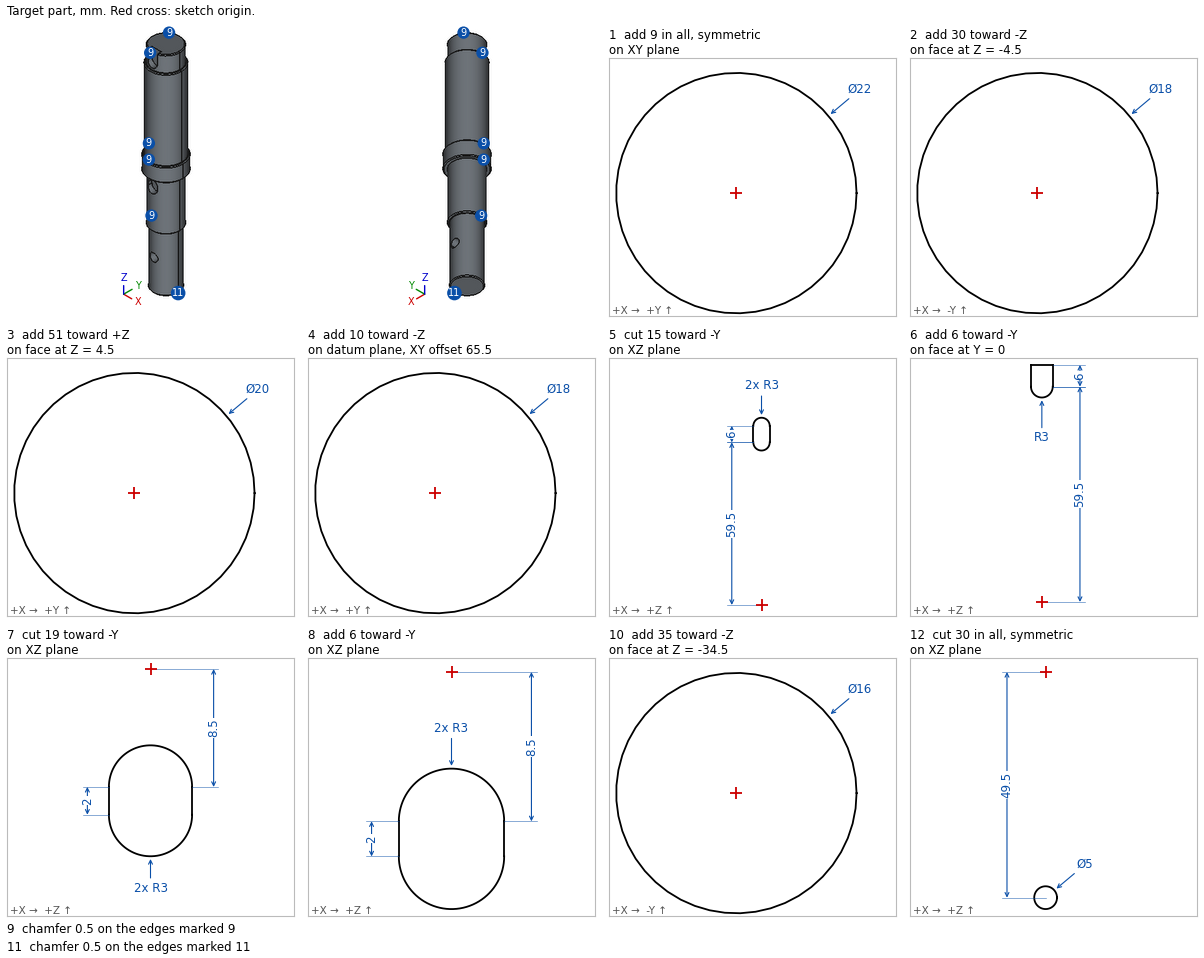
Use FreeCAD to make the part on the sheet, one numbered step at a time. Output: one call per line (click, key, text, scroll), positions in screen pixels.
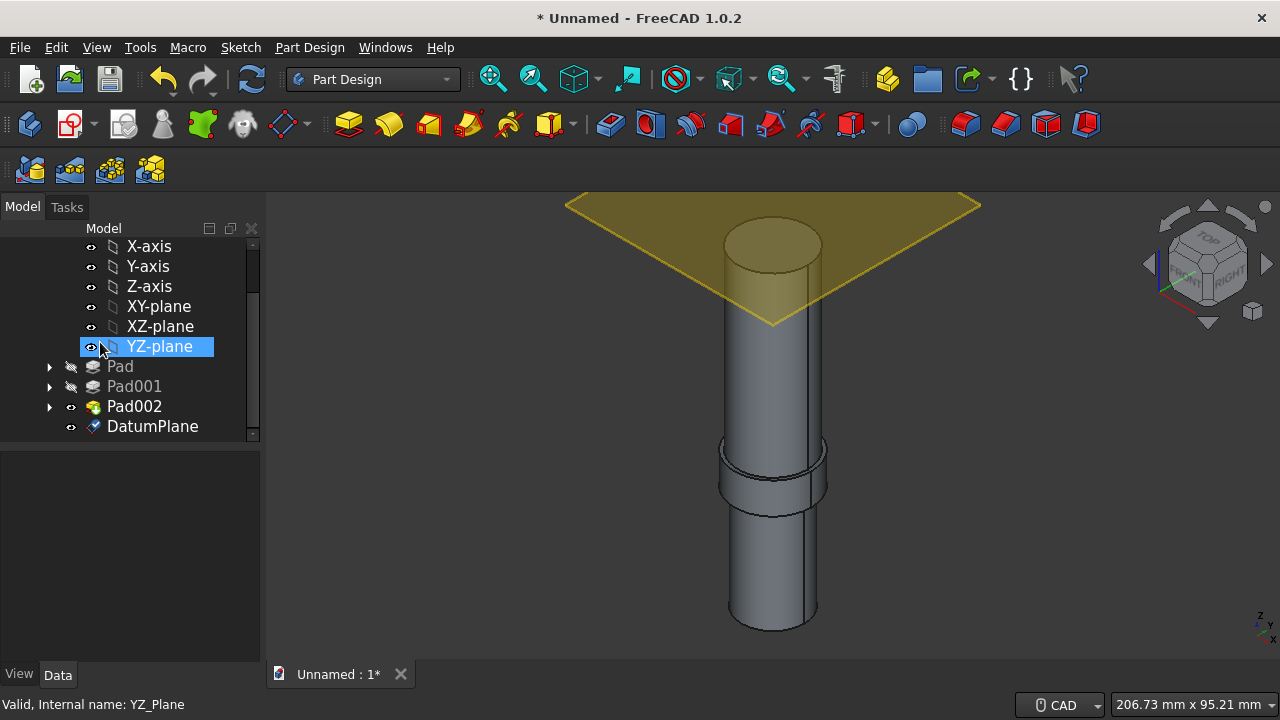
click(116, 427)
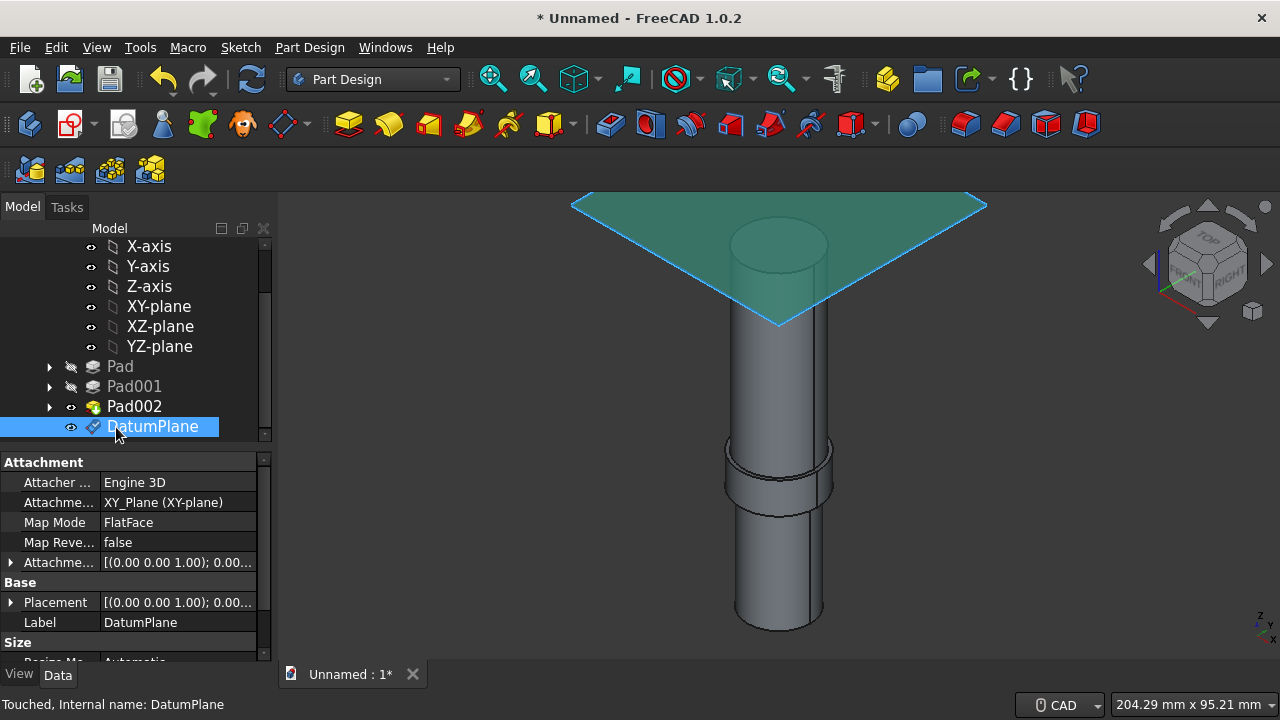
click(70, 124)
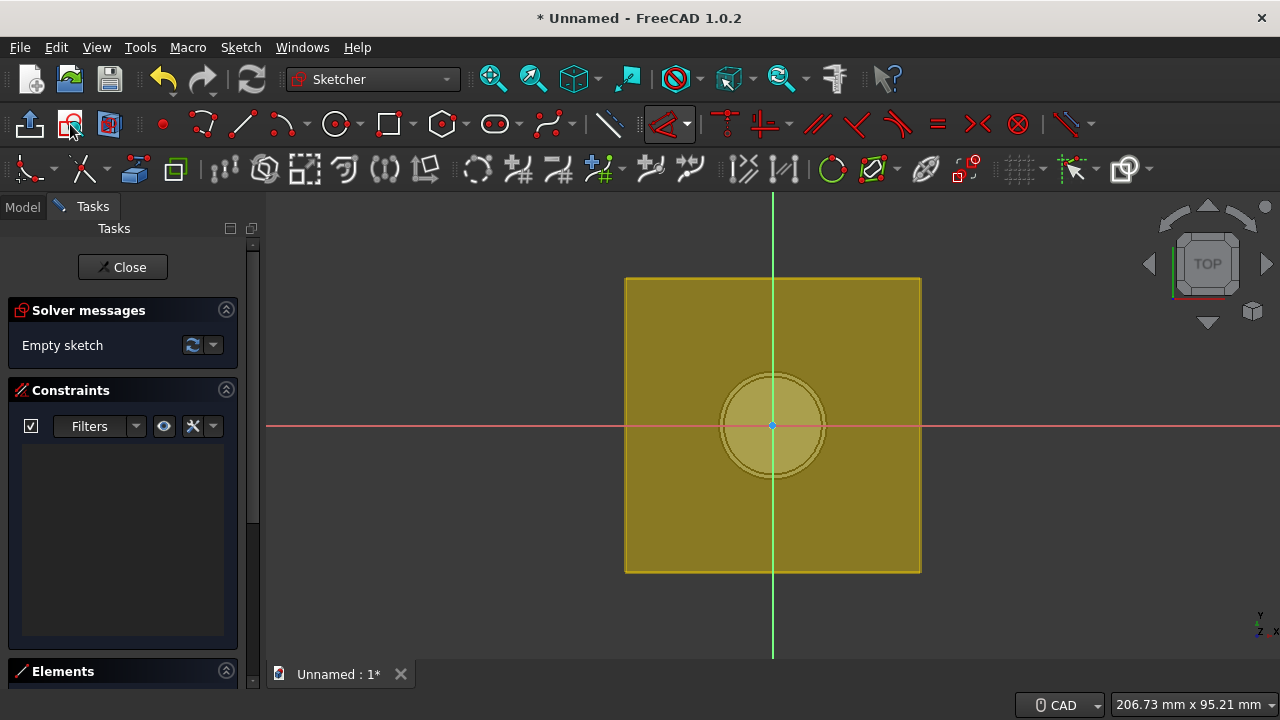
scroll(802, 426, up, 6)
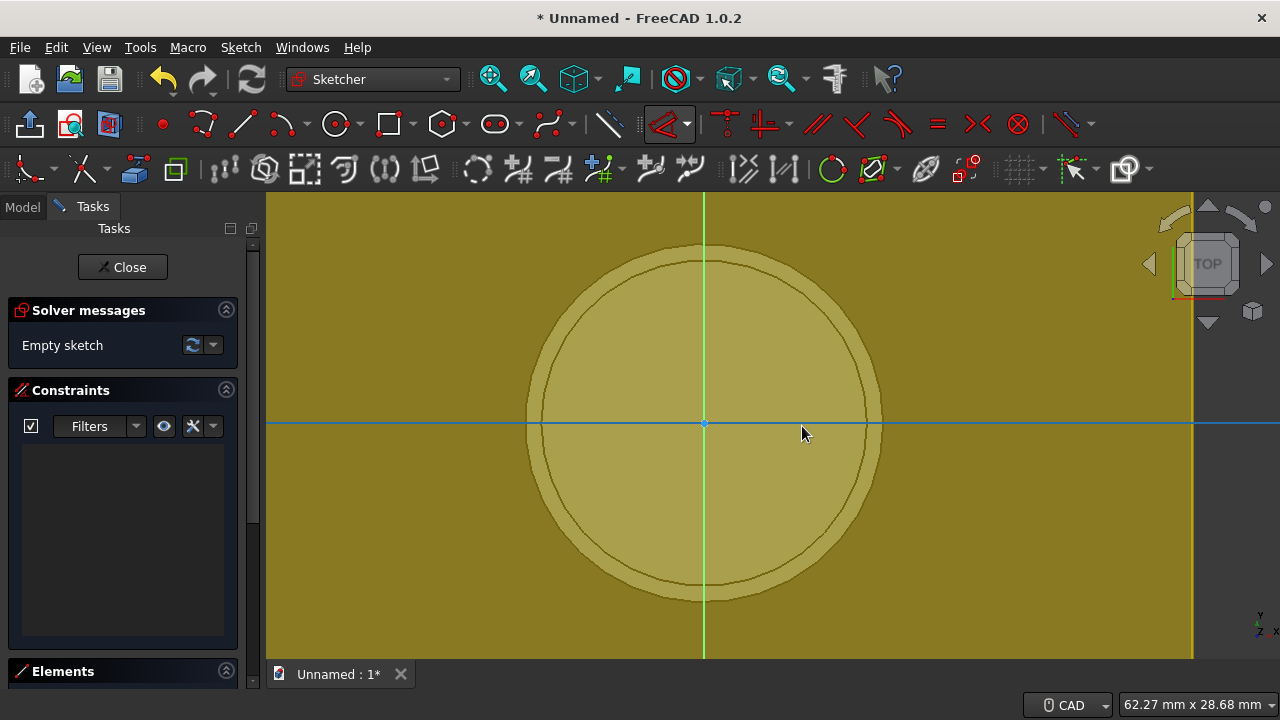
click(336, 124)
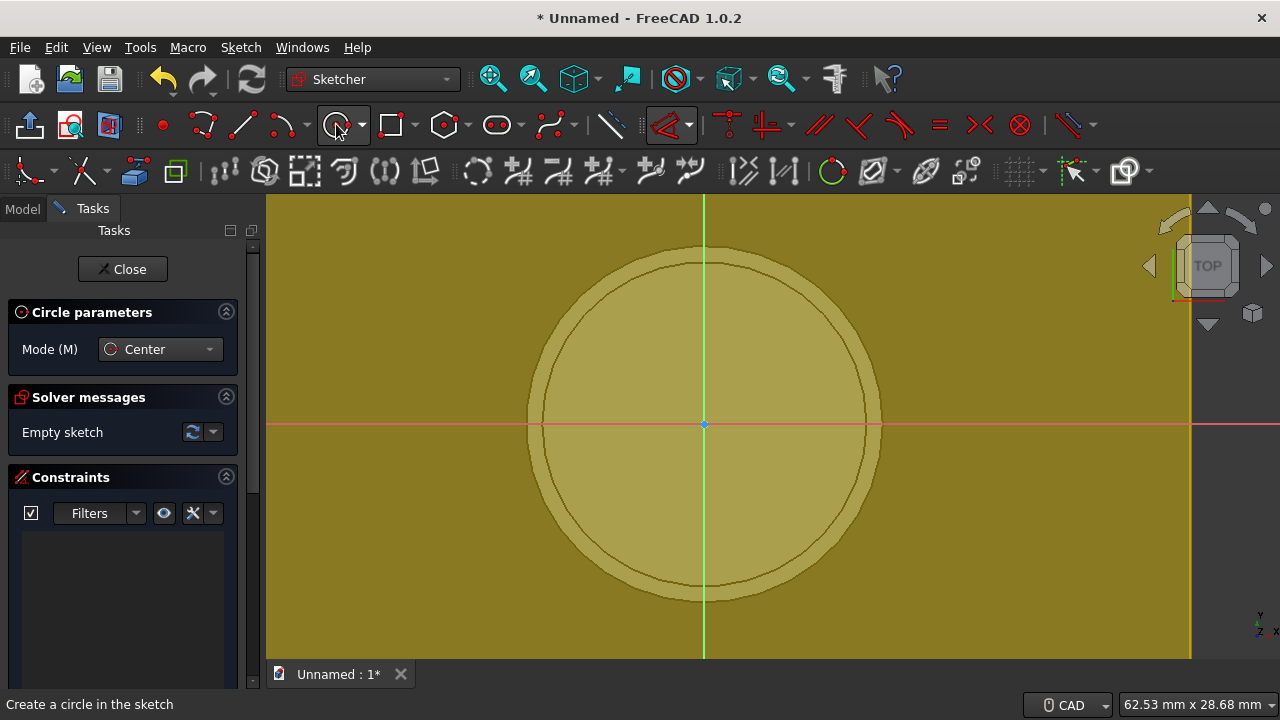
click(704, 424)
click(808, 321)
key(Escape)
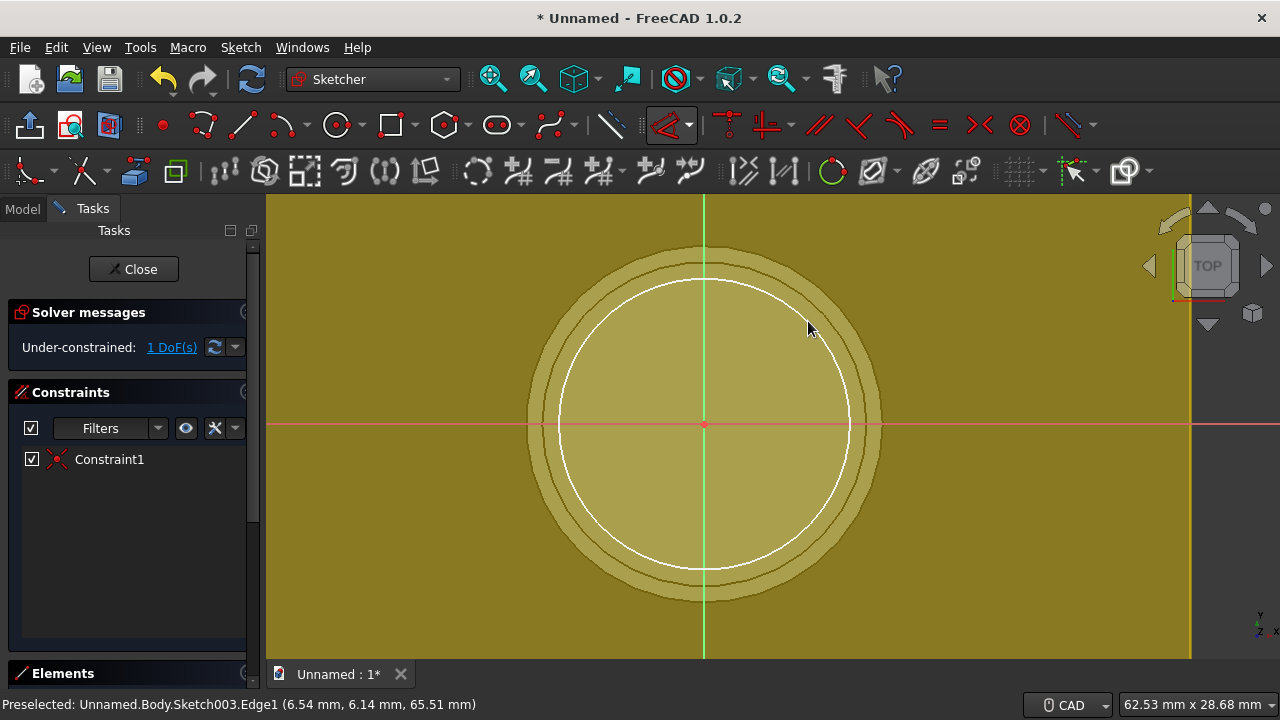
click(807, 321)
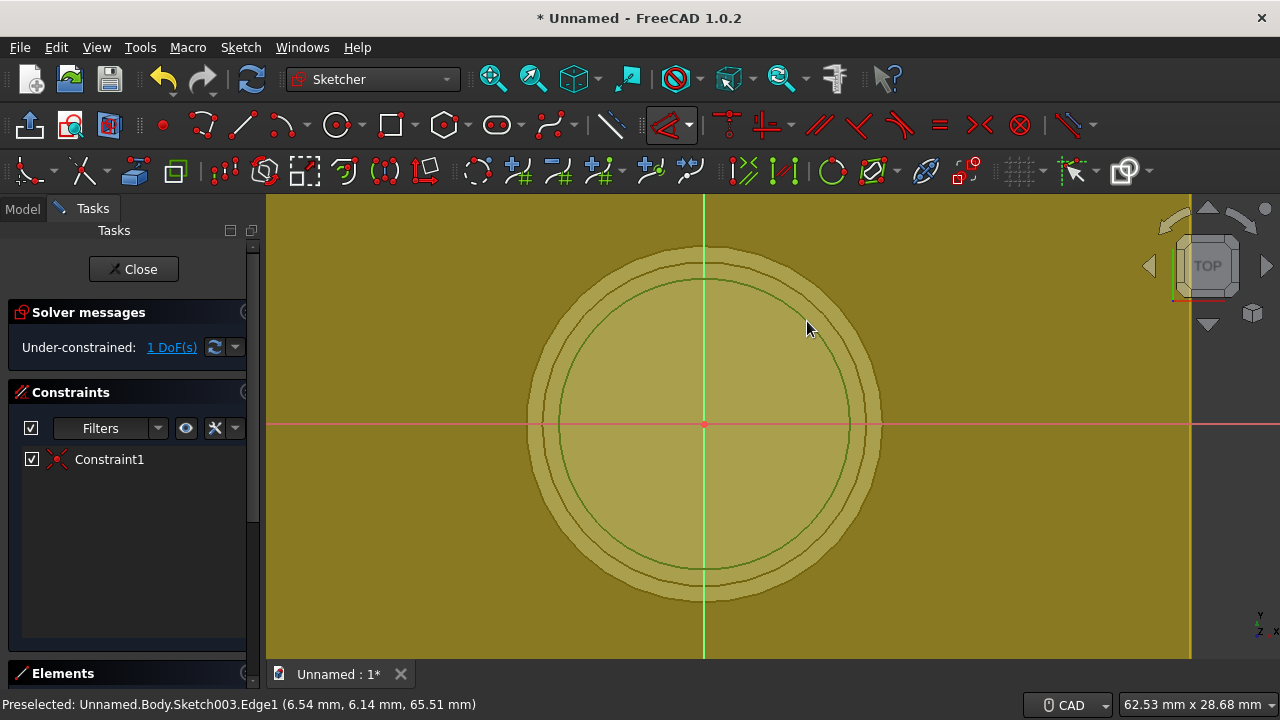
click(692, 126)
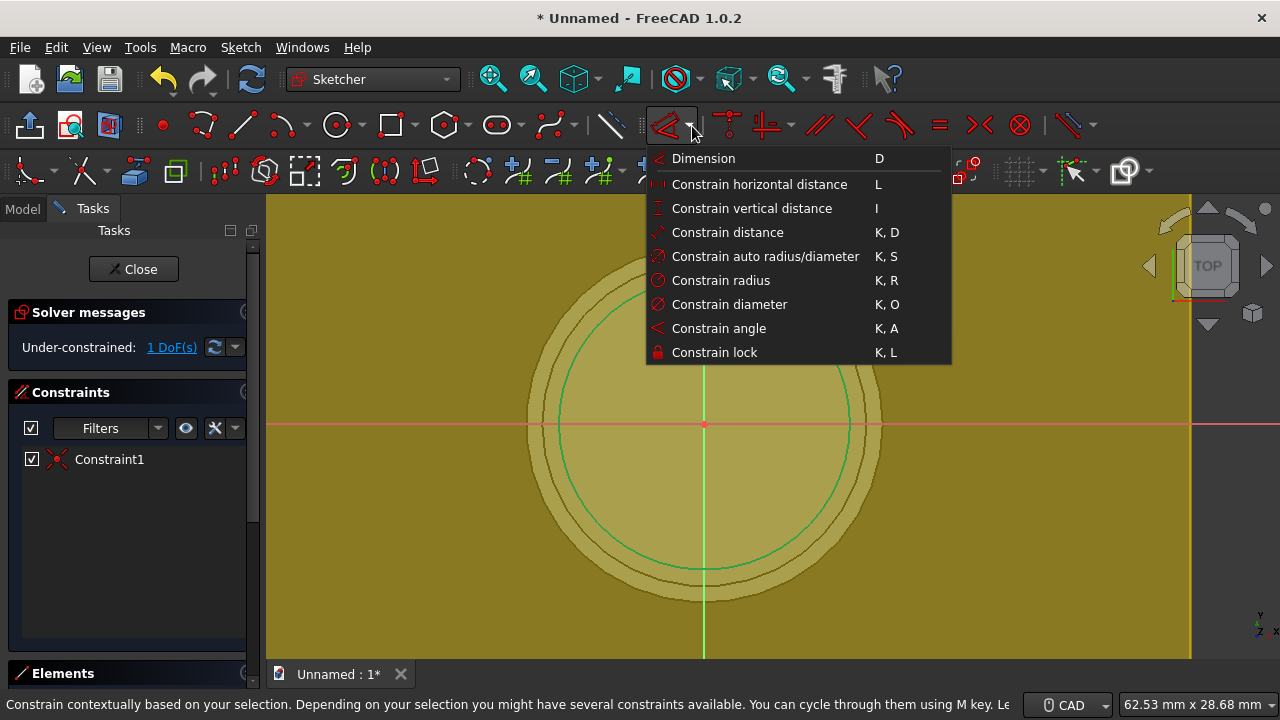
click(799, 304)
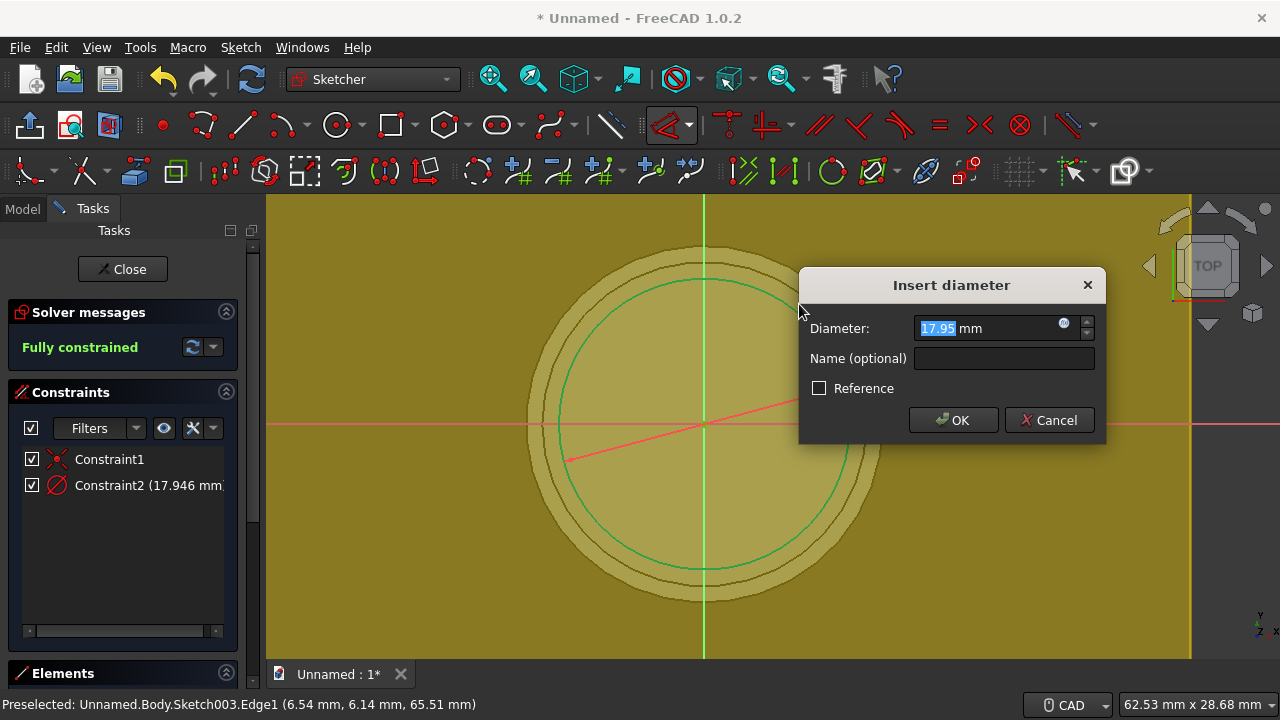
text(18)
key(Return)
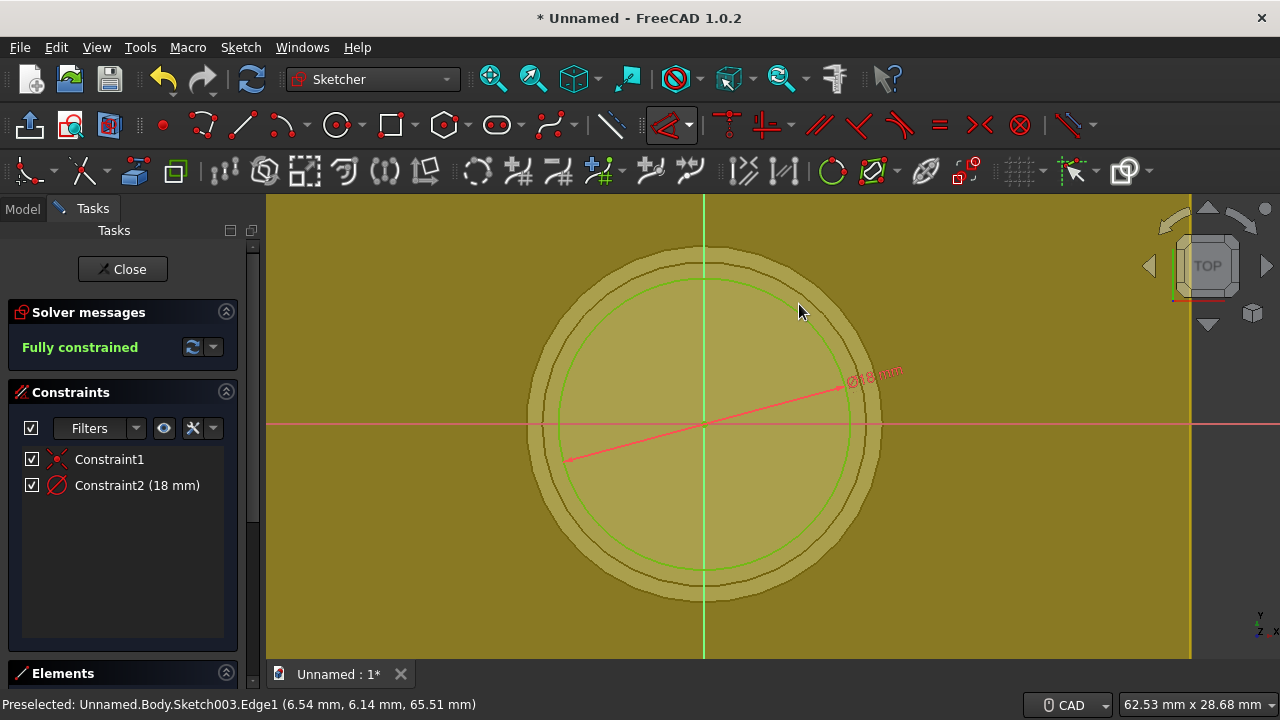
click(123, 269)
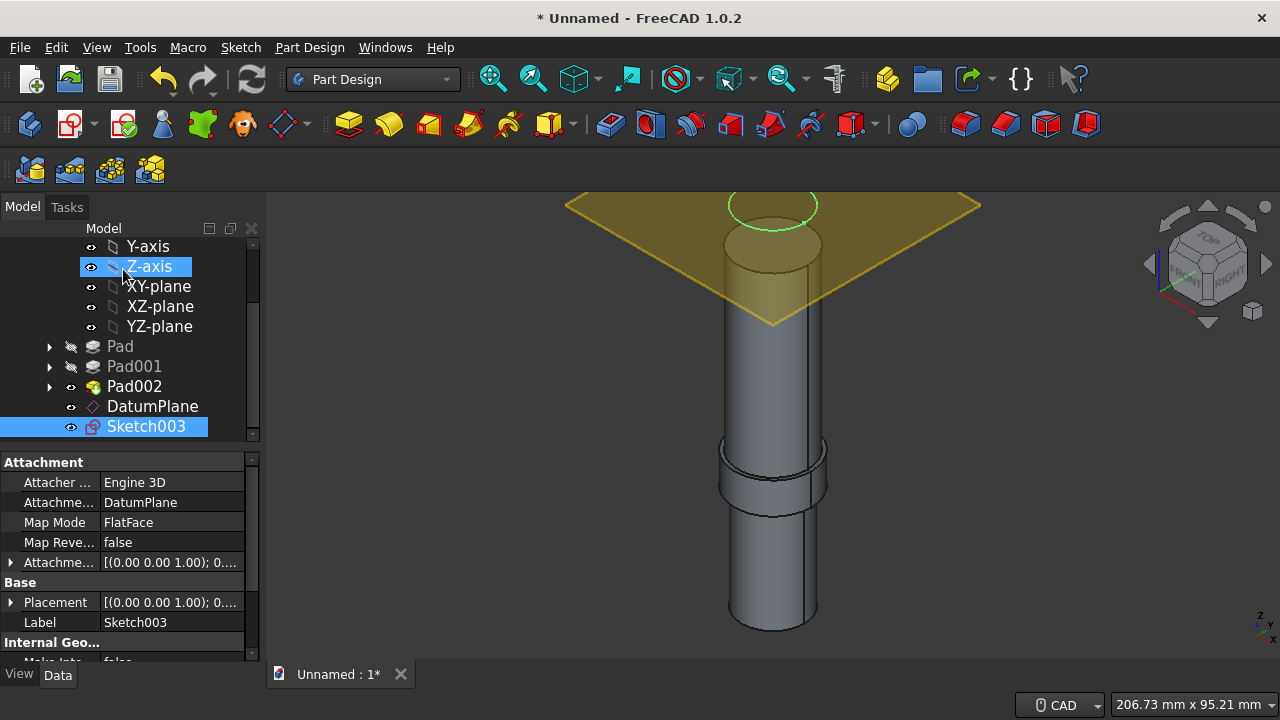
click(350, 124)